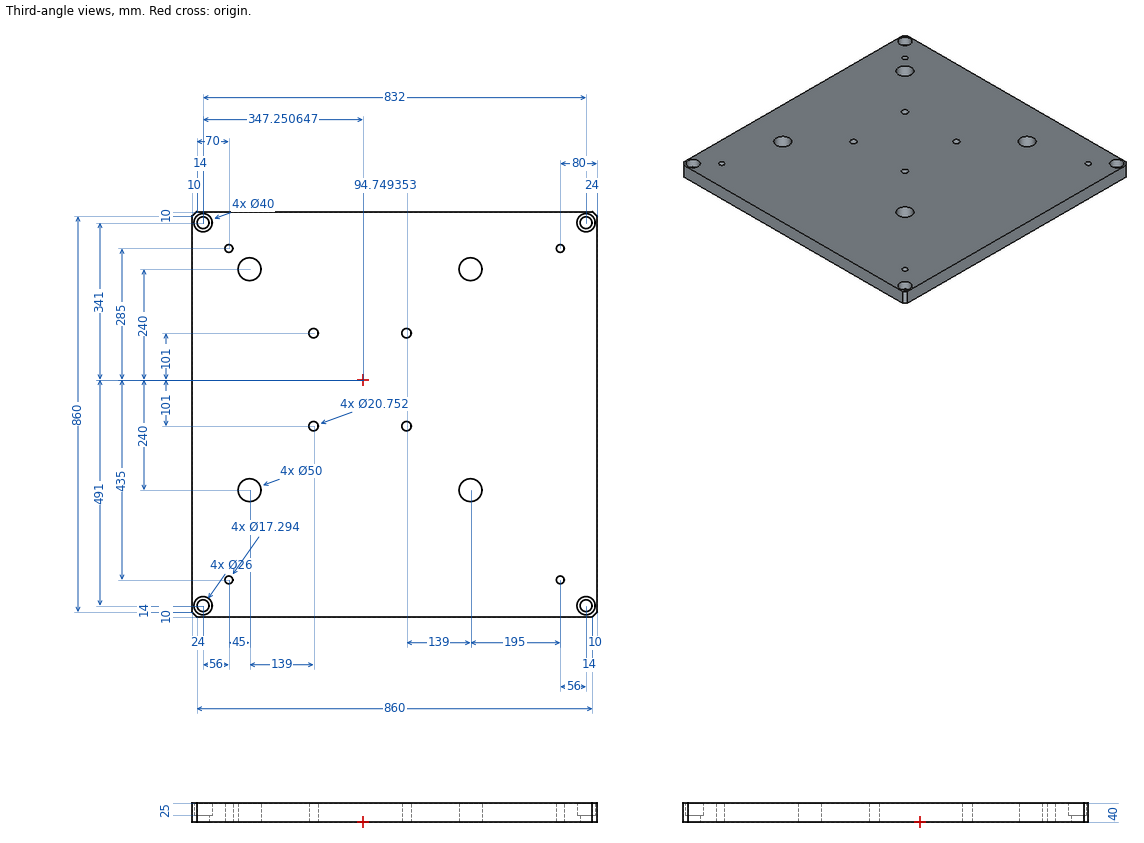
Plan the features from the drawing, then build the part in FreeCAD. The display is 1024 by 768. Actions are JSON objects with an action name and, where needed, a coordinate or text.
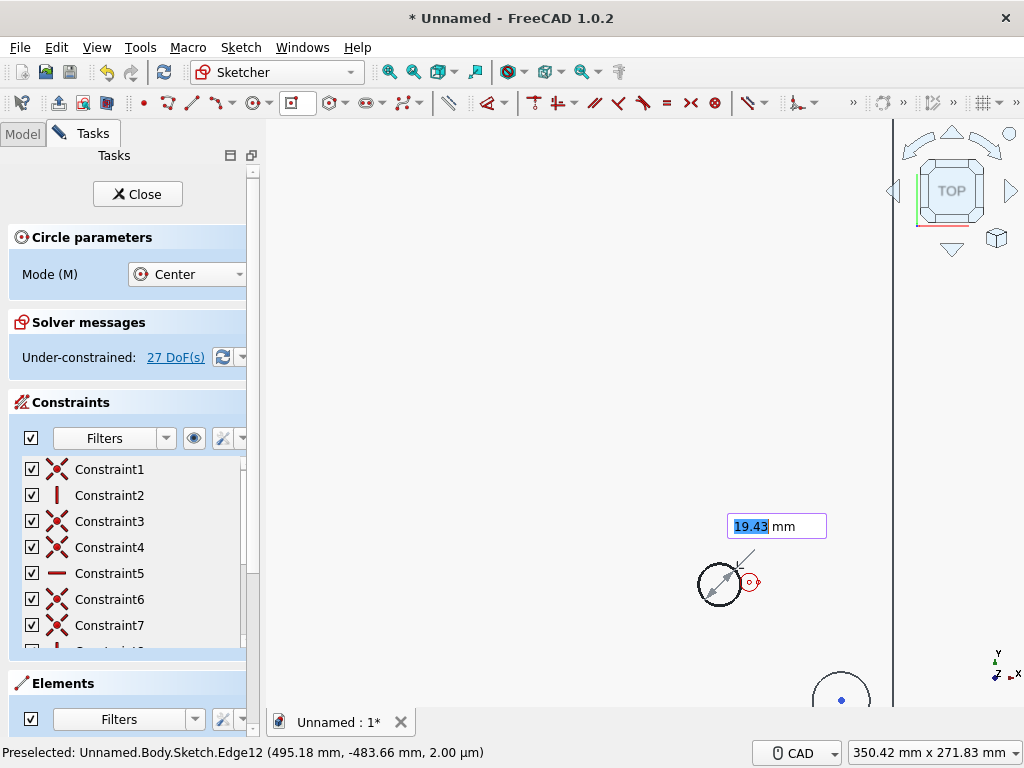
{"action": "left_click", "coordinate": [734, 565]}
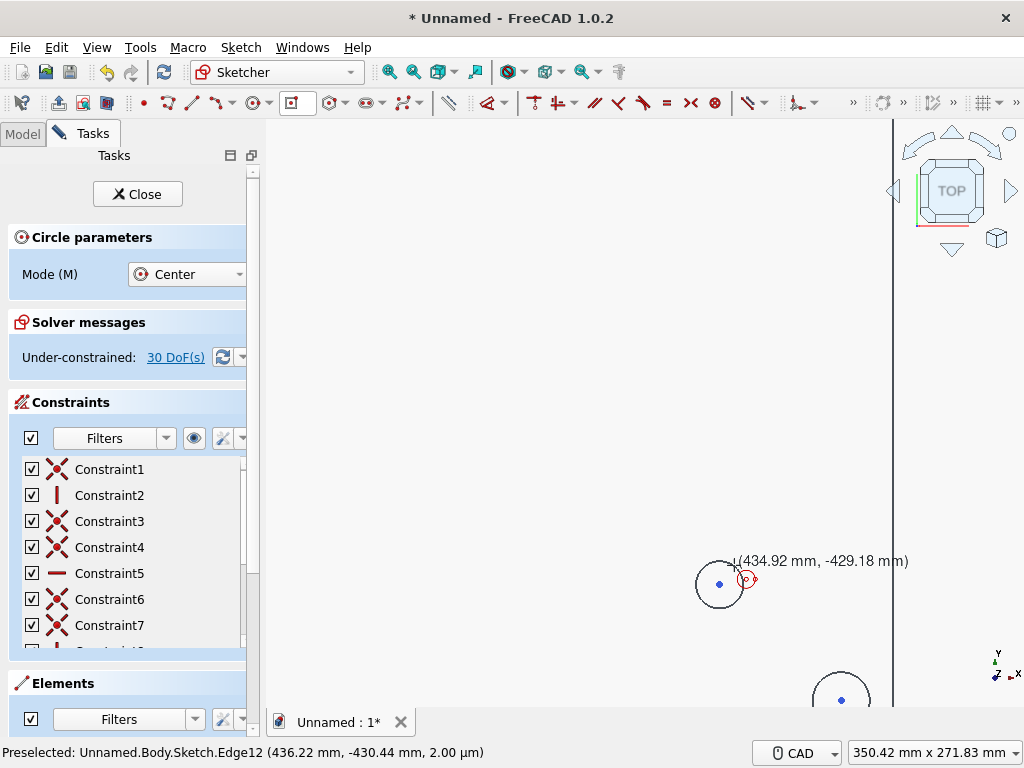
{"action": "scroll", "coordinate": [737, 568], "scroll_direction": "down", "scroll_amount": 8}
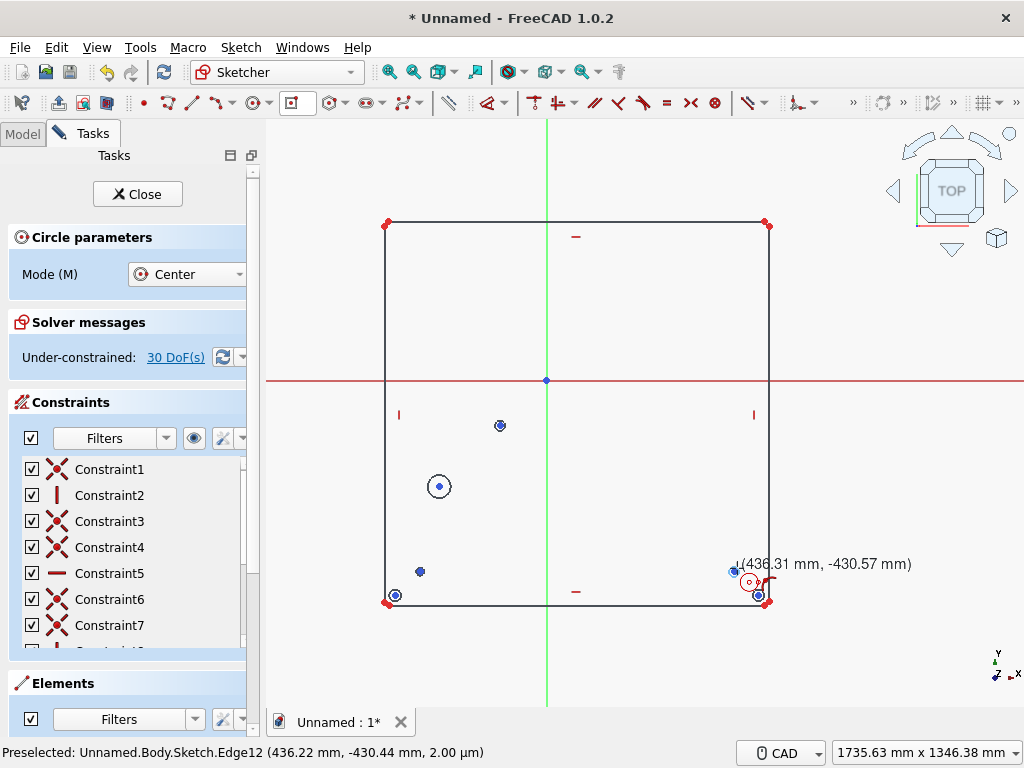
{"action": "left_click", "coordinate": [649, 486]}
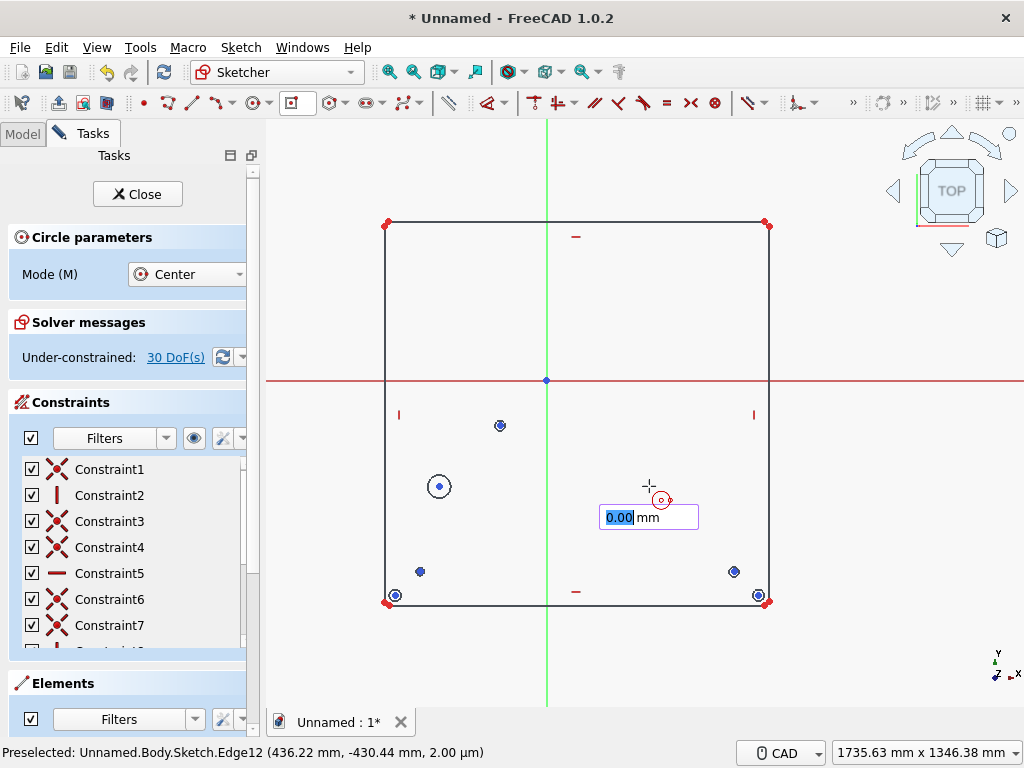
{"action": "scroll", "coordinate": [657, 478], "scroll_direction": "up", "scroll_amount": 2}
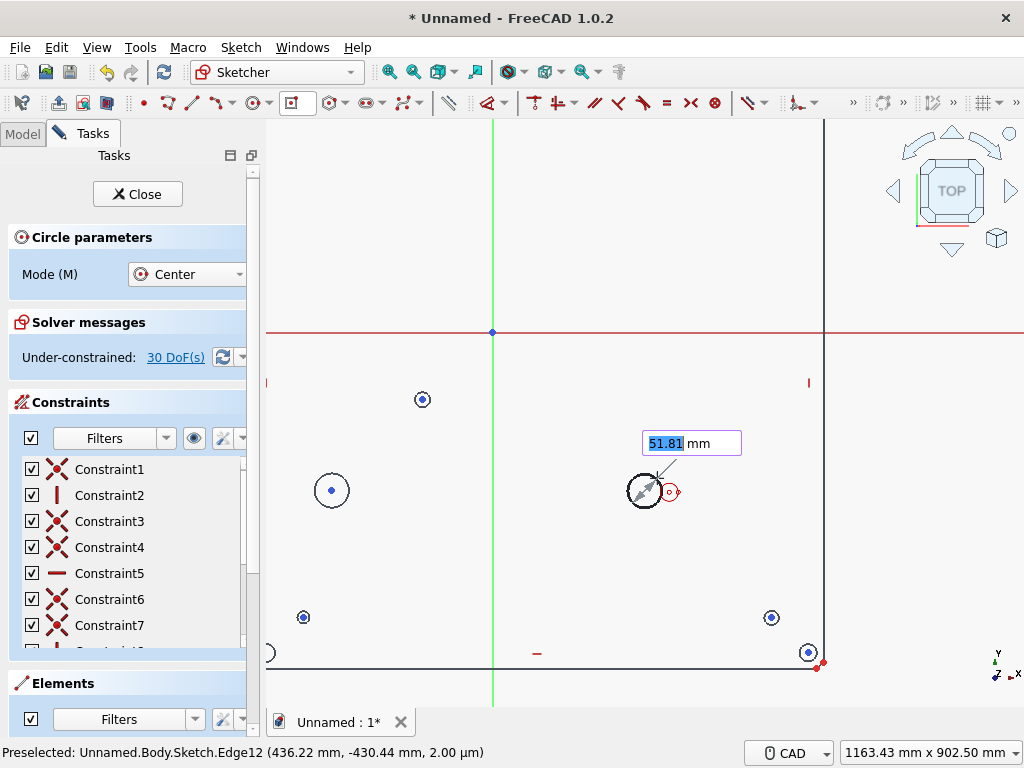
{"action": "left_click", "coordinate": [656, 477]}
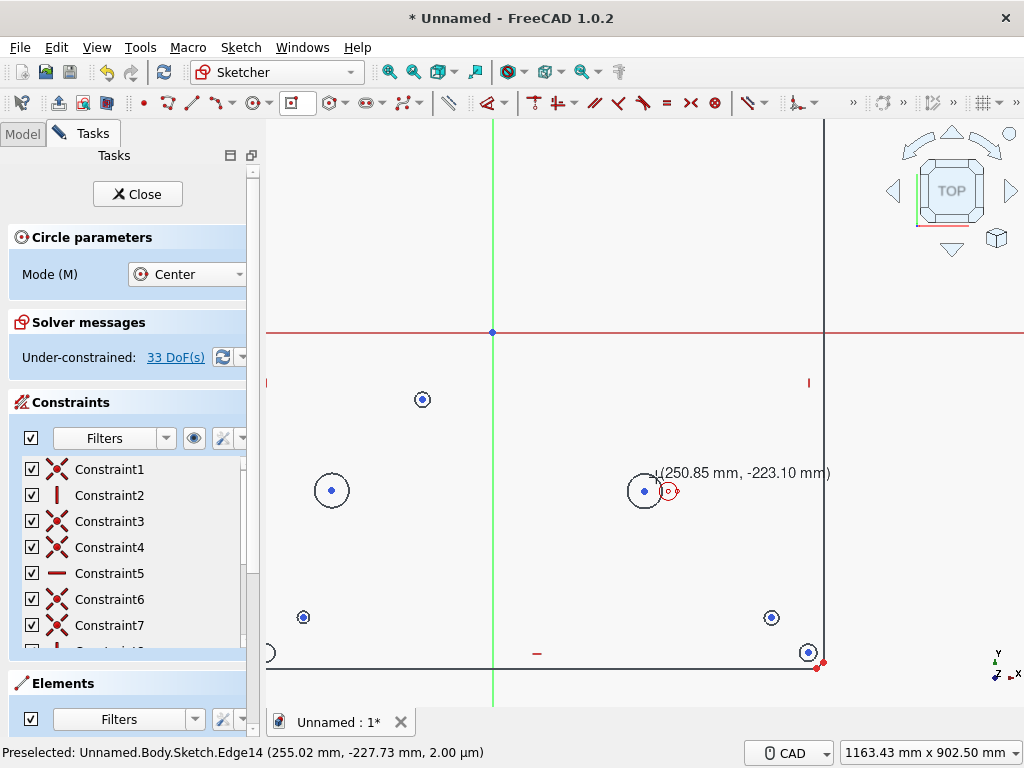
{"action": "scroll", "coordinate": [554, 398], "scroll_direction": "up", "scroll_amount": 7}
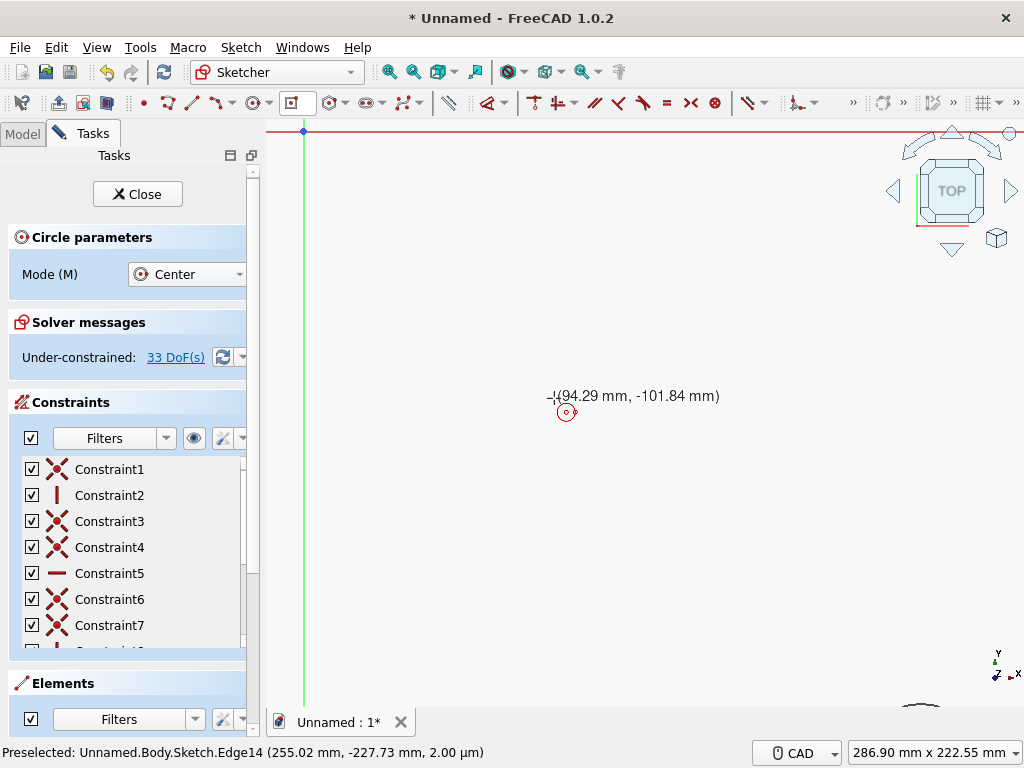
{"action": "scroll", "coordinate": [595, 429], "scroll_direction": "down", "scroll_amount": 9}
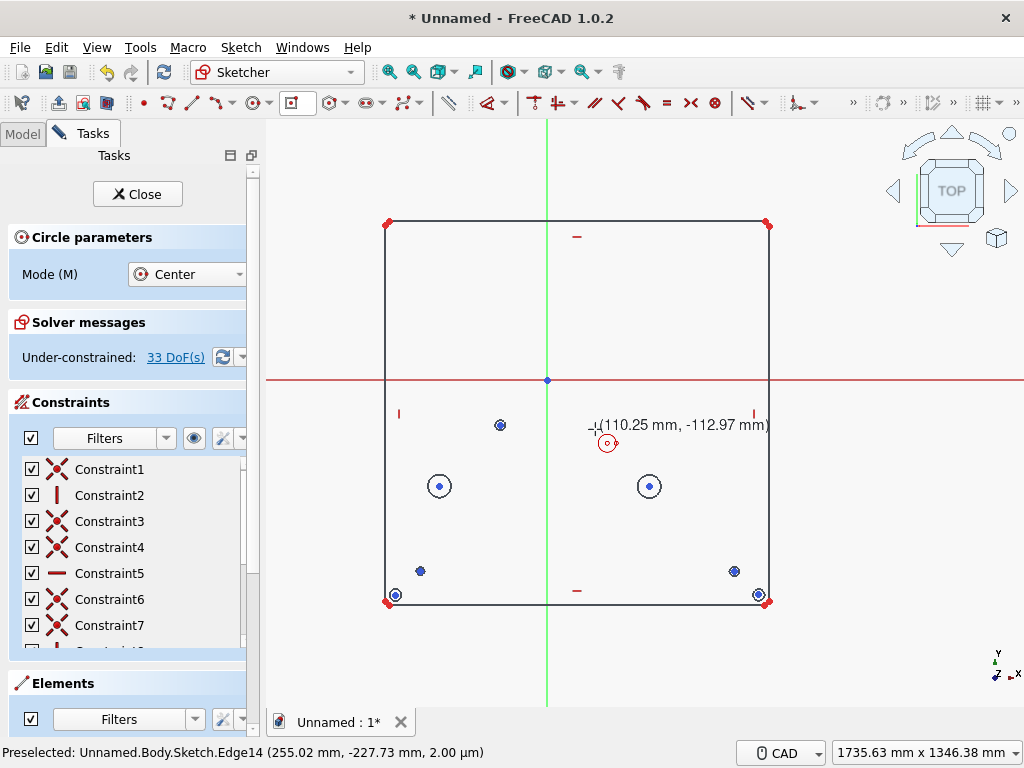
{"action": "left_click", "coordinate": [589, 424]}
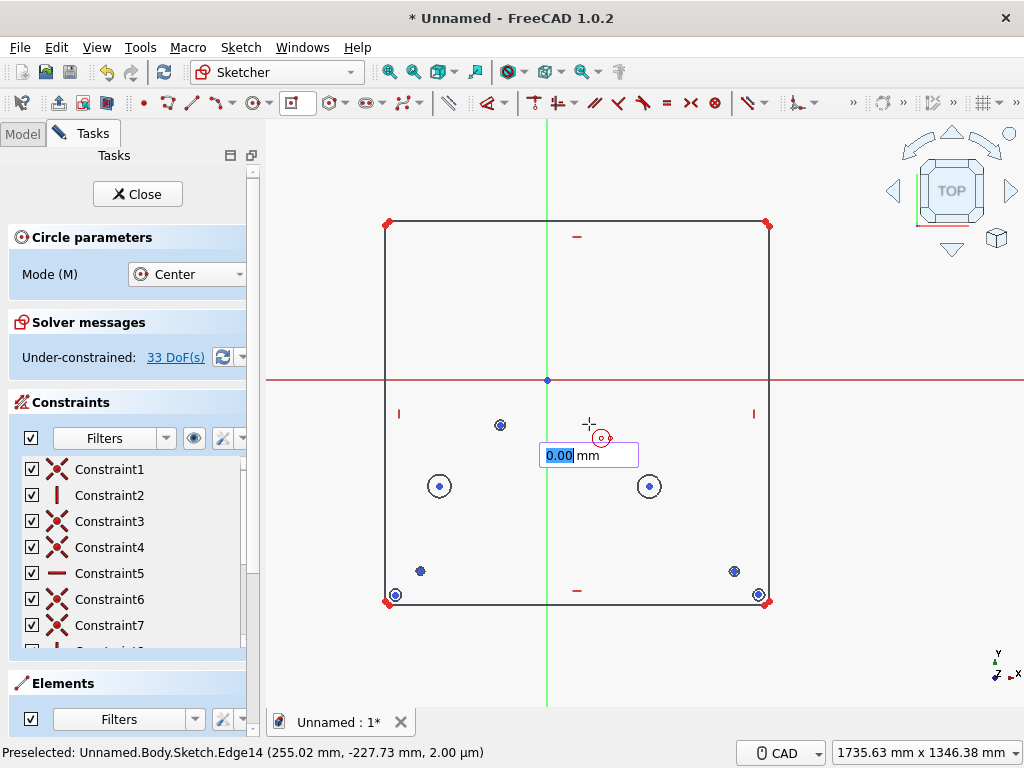
{"action": "scroll", "coordinate": [592, 421], "scroll_direction": "up", "scroll_amount": 7}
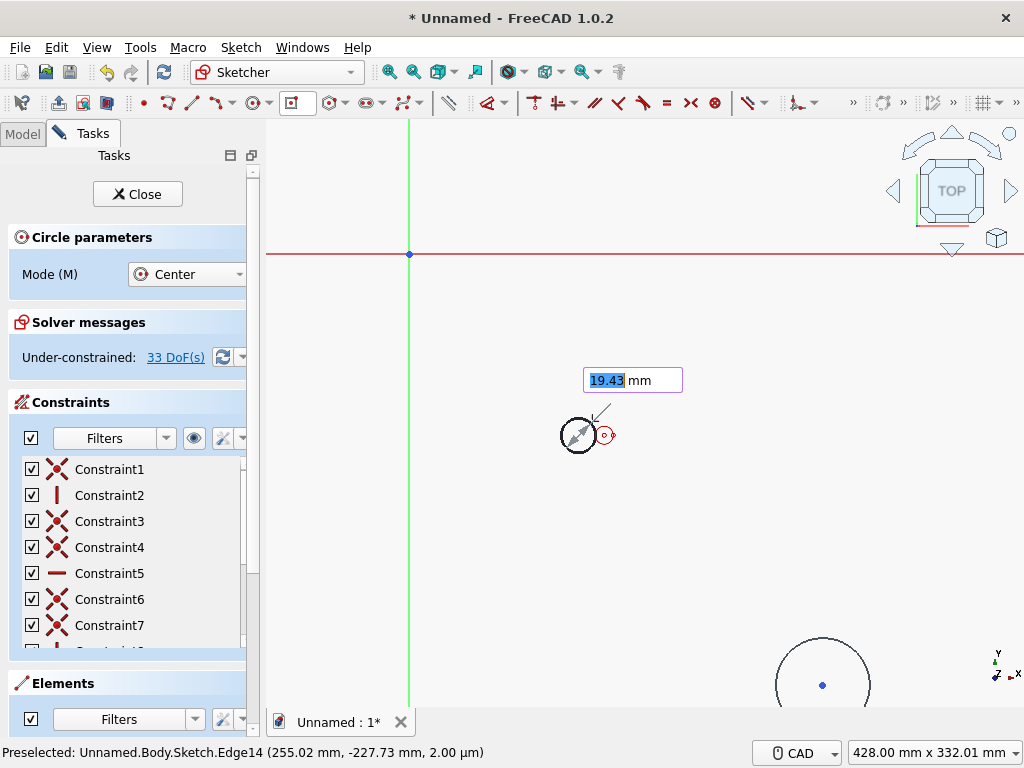
{"action": "left_click", "coordinate": [590, 420]}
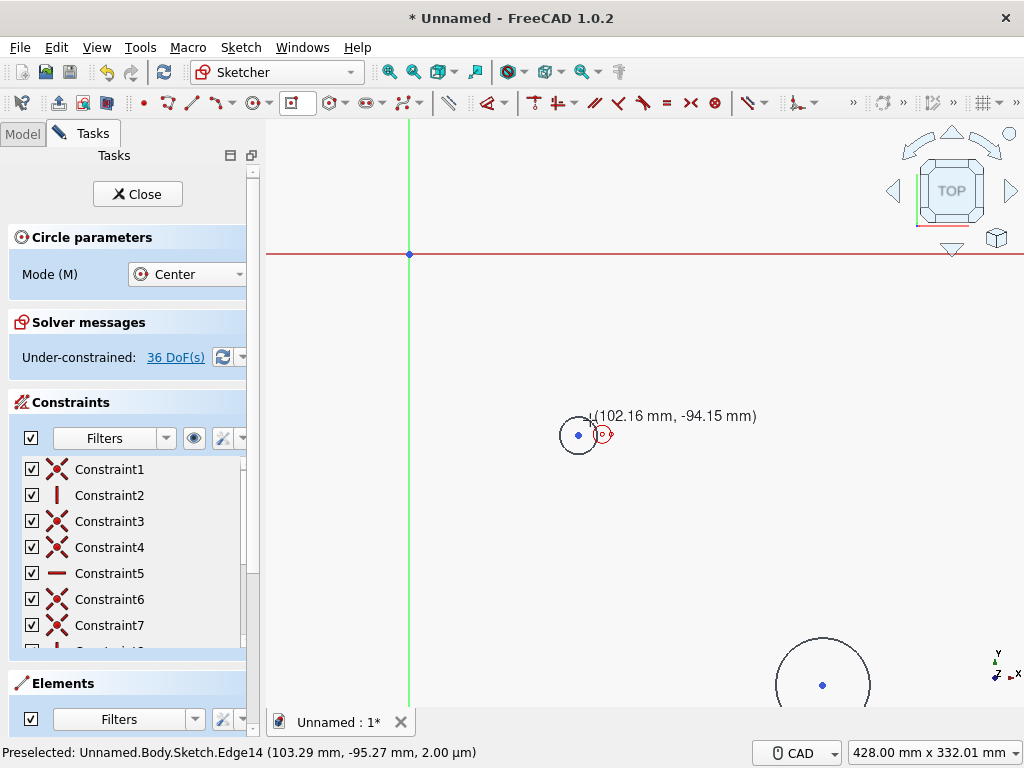
{"action": "scroll", "coordinate": [591, 421], "scroll_direction": "down", "scroll_amount": 7}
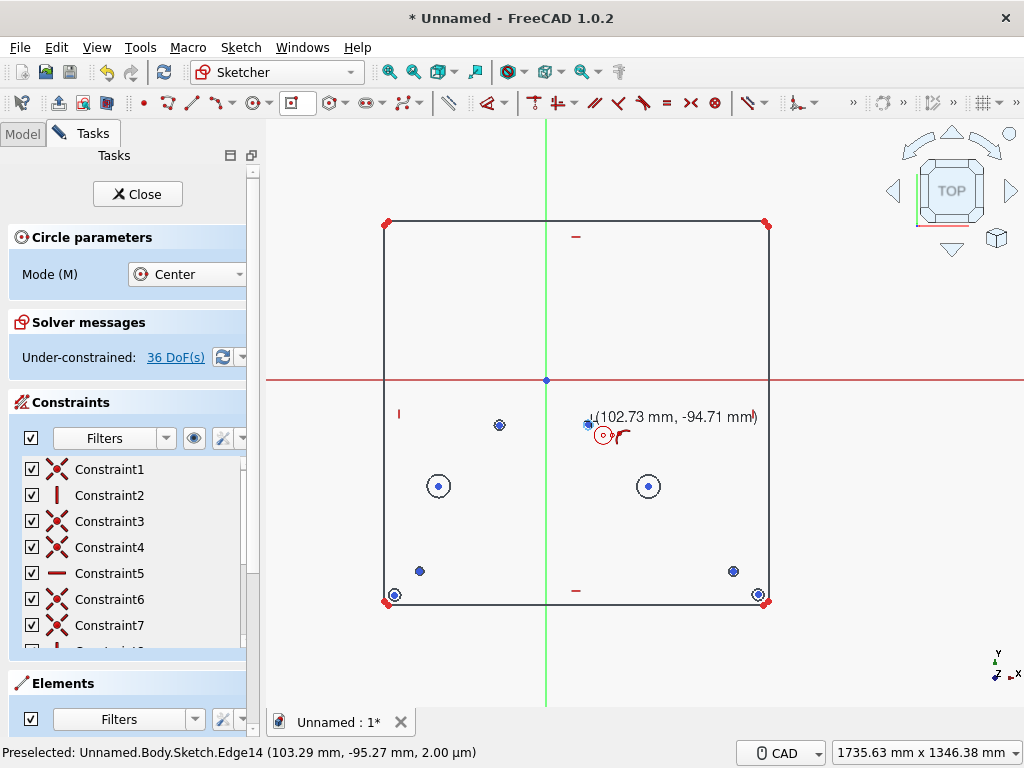
{"action": "scroll", "coordinate": [500, 336], "scroll_direction": "up", "scroll_amount": 9}